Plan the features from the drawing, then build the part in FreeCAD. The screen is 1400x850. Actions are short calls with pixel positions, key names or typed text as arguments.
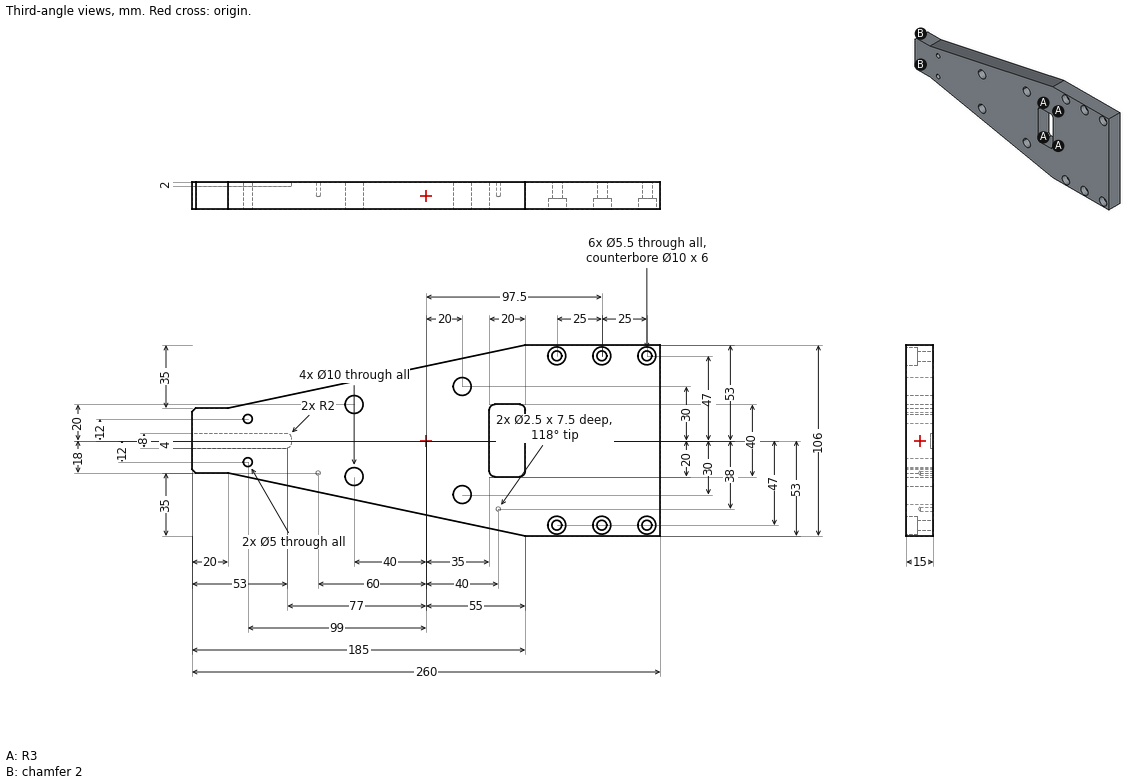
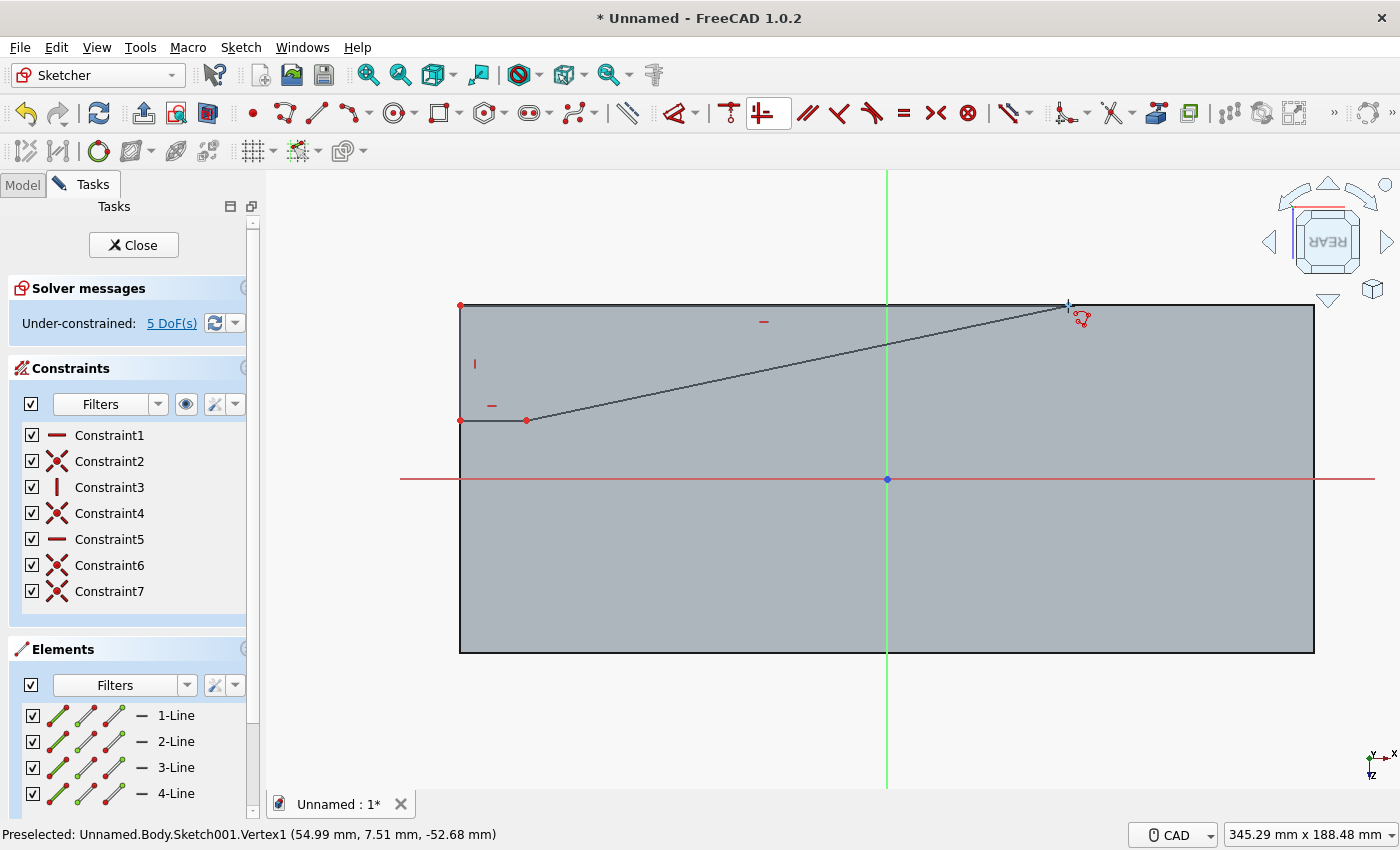
click(1068, 653)
click(526, 538)
click(460, 538)
click(460, 653)
click(1068, 654)
key(Escape)
key(Escape)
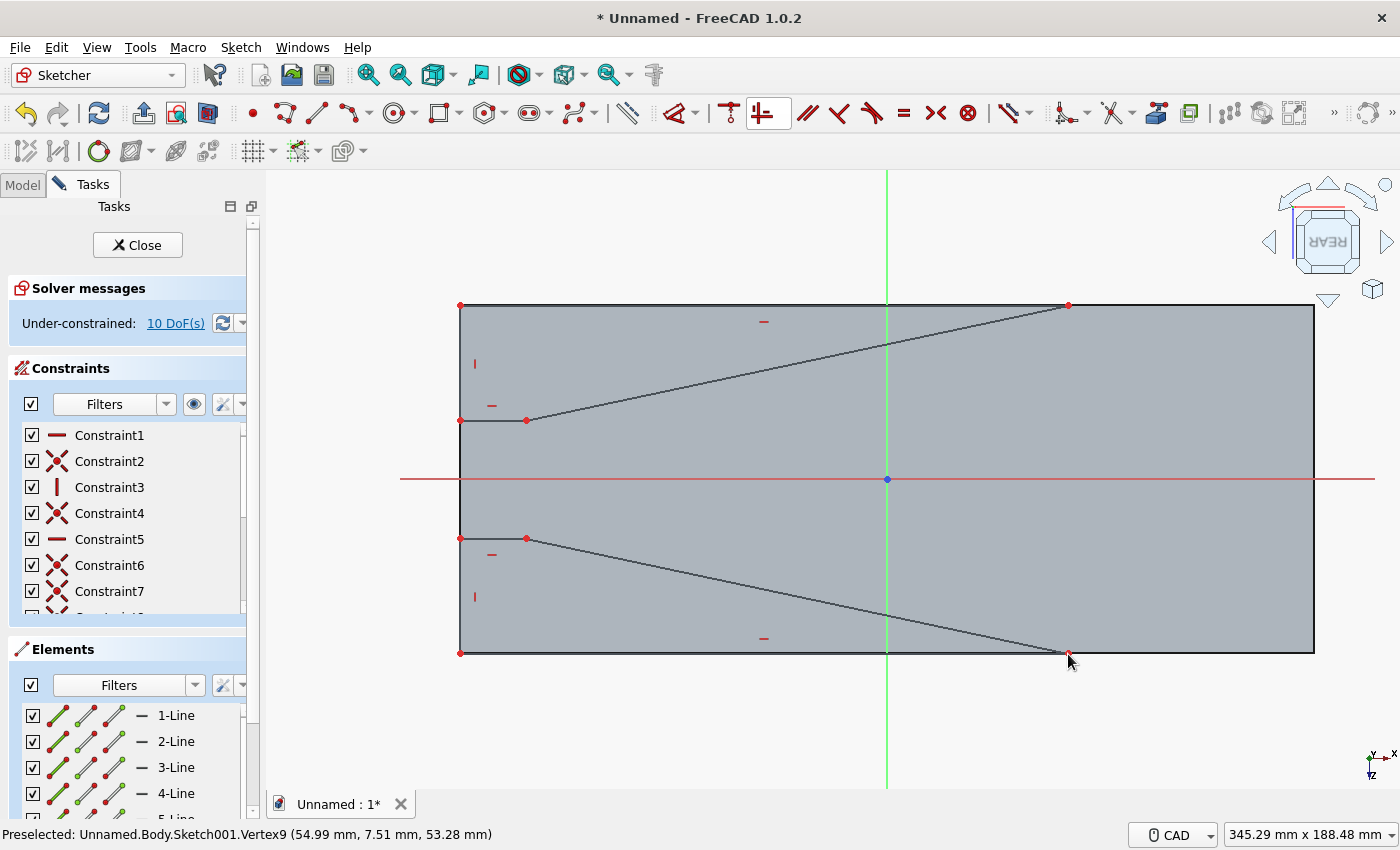
key(d)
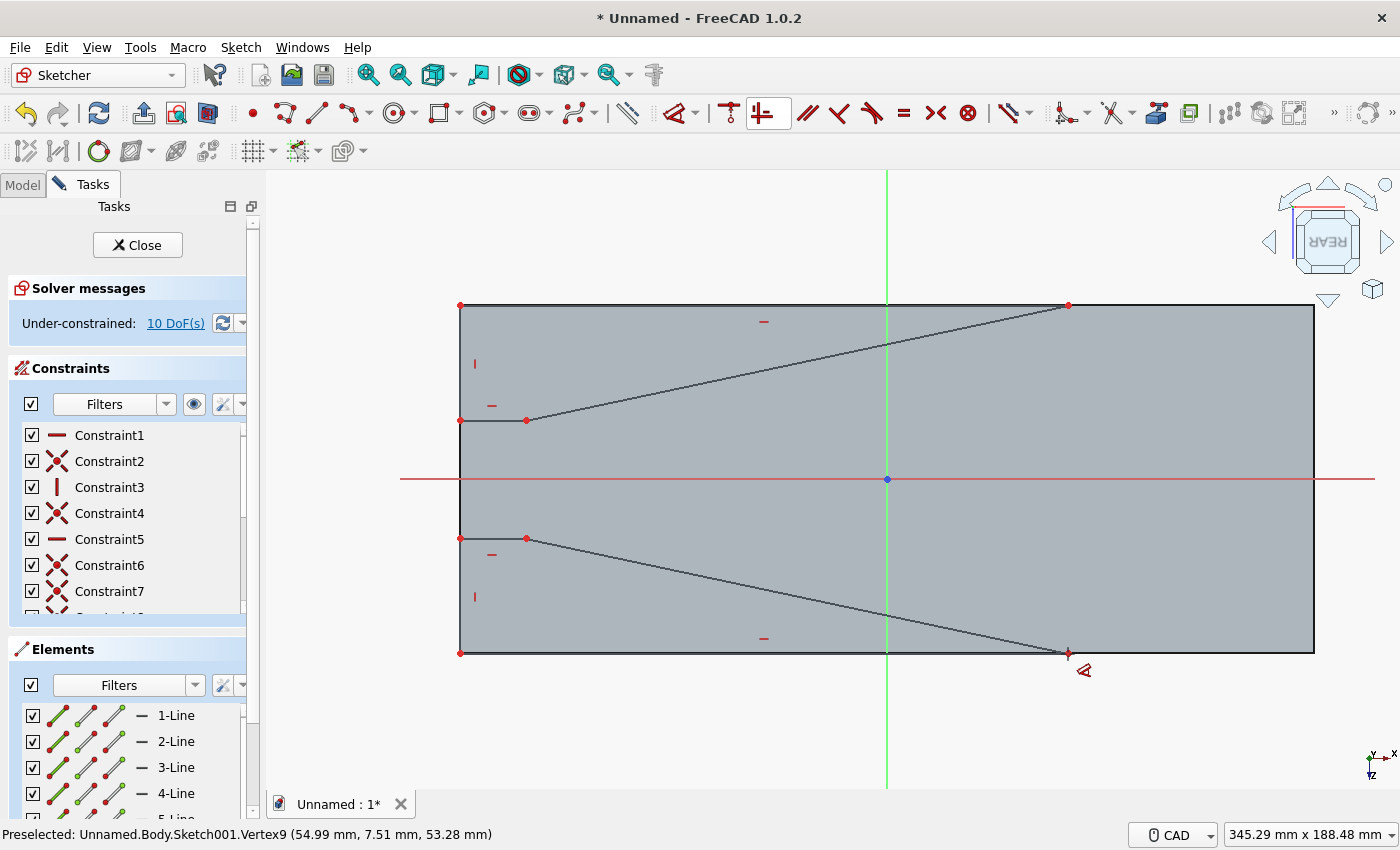
click(460, 341)
click(426, 364)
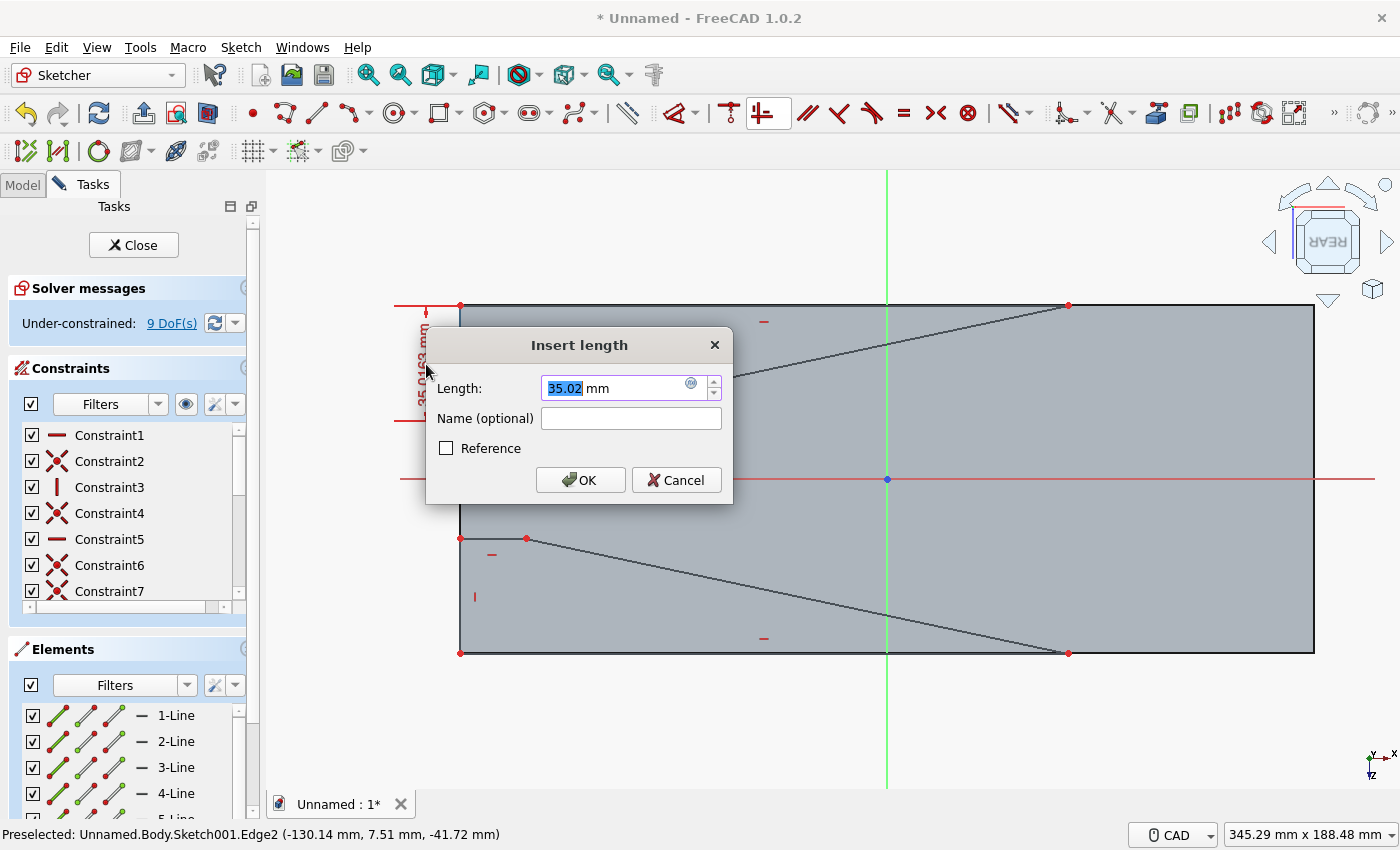
text(35)
key(Return)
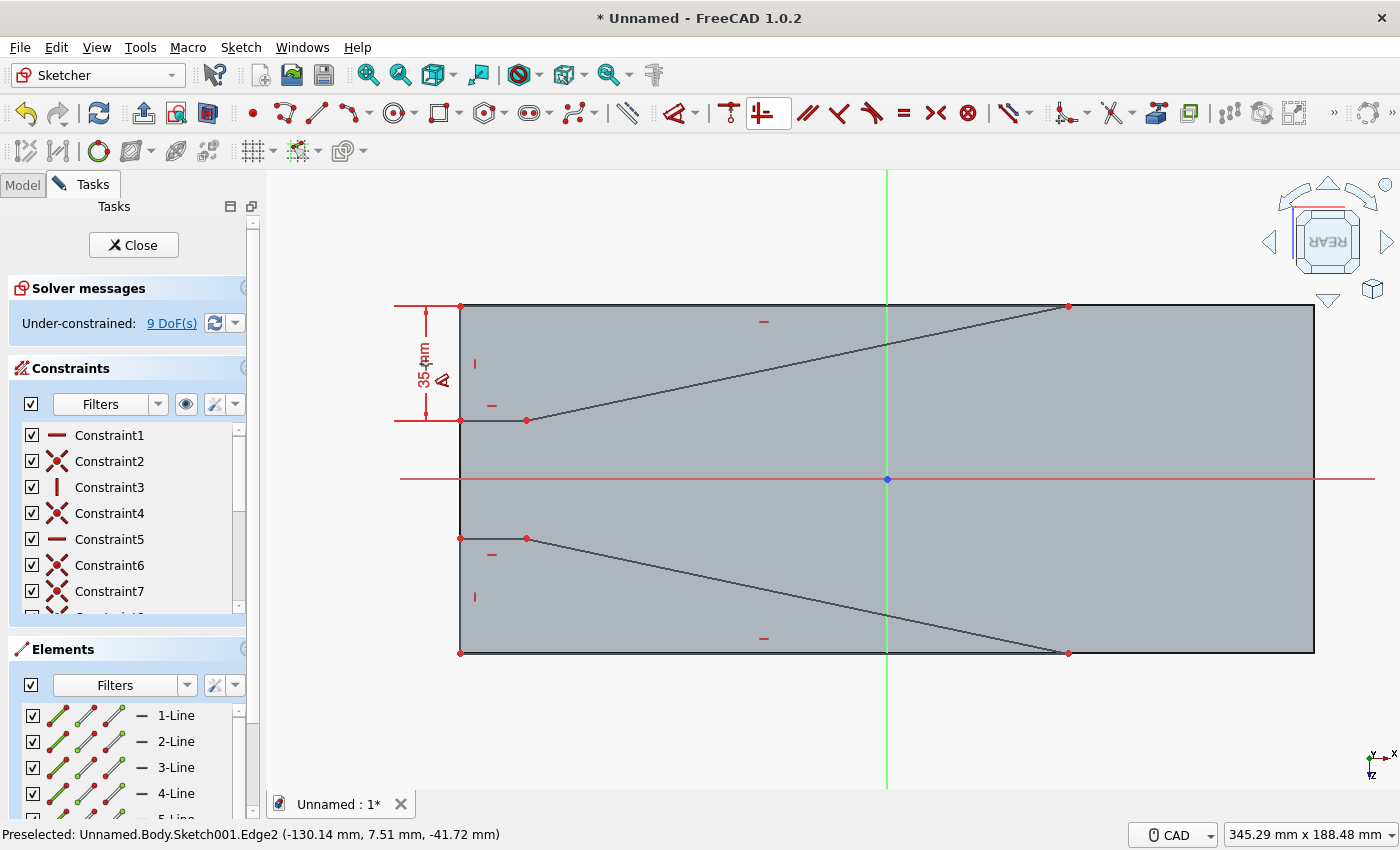
click(480, 421)
click(493, 387)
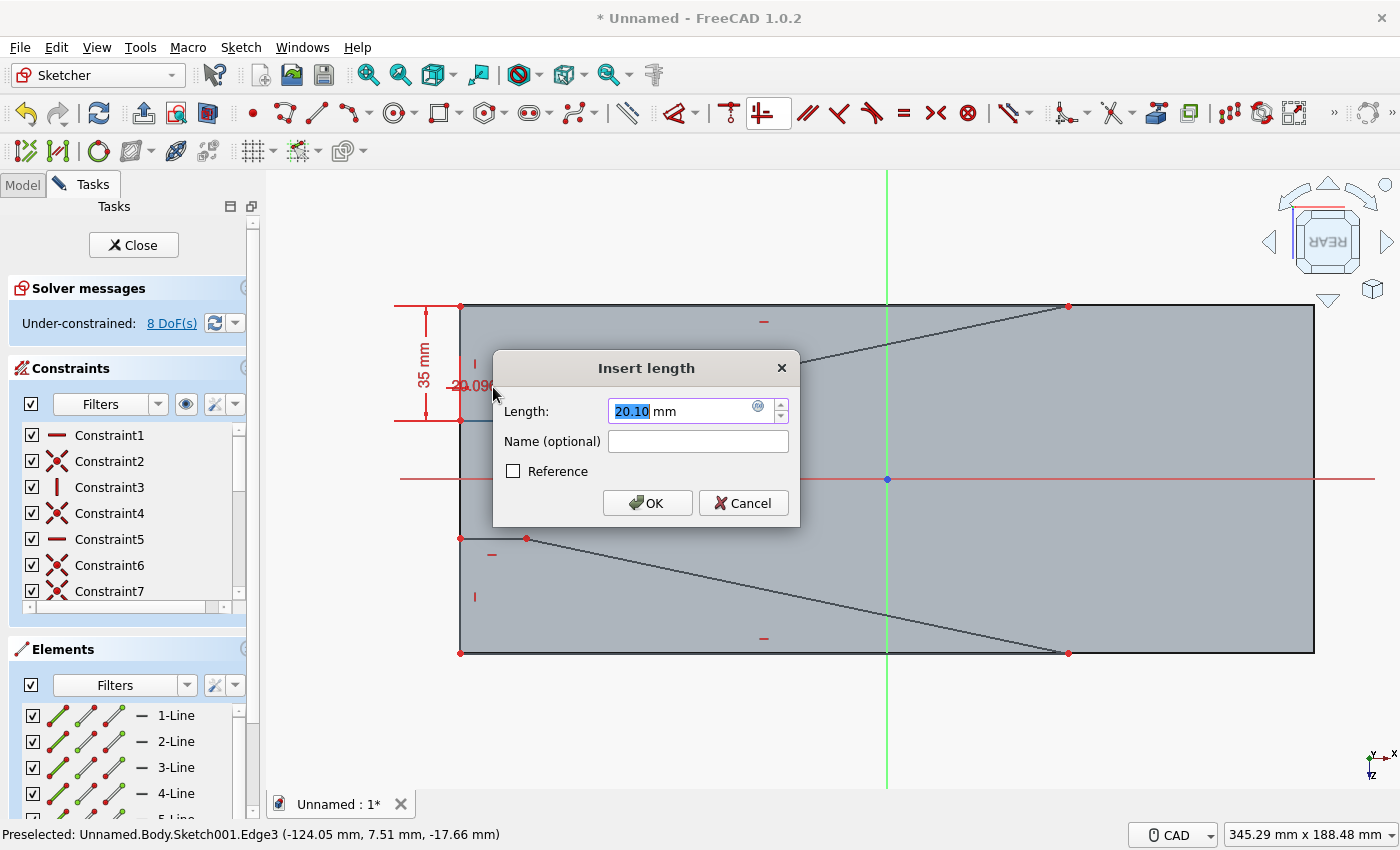
text(20)
key(Return)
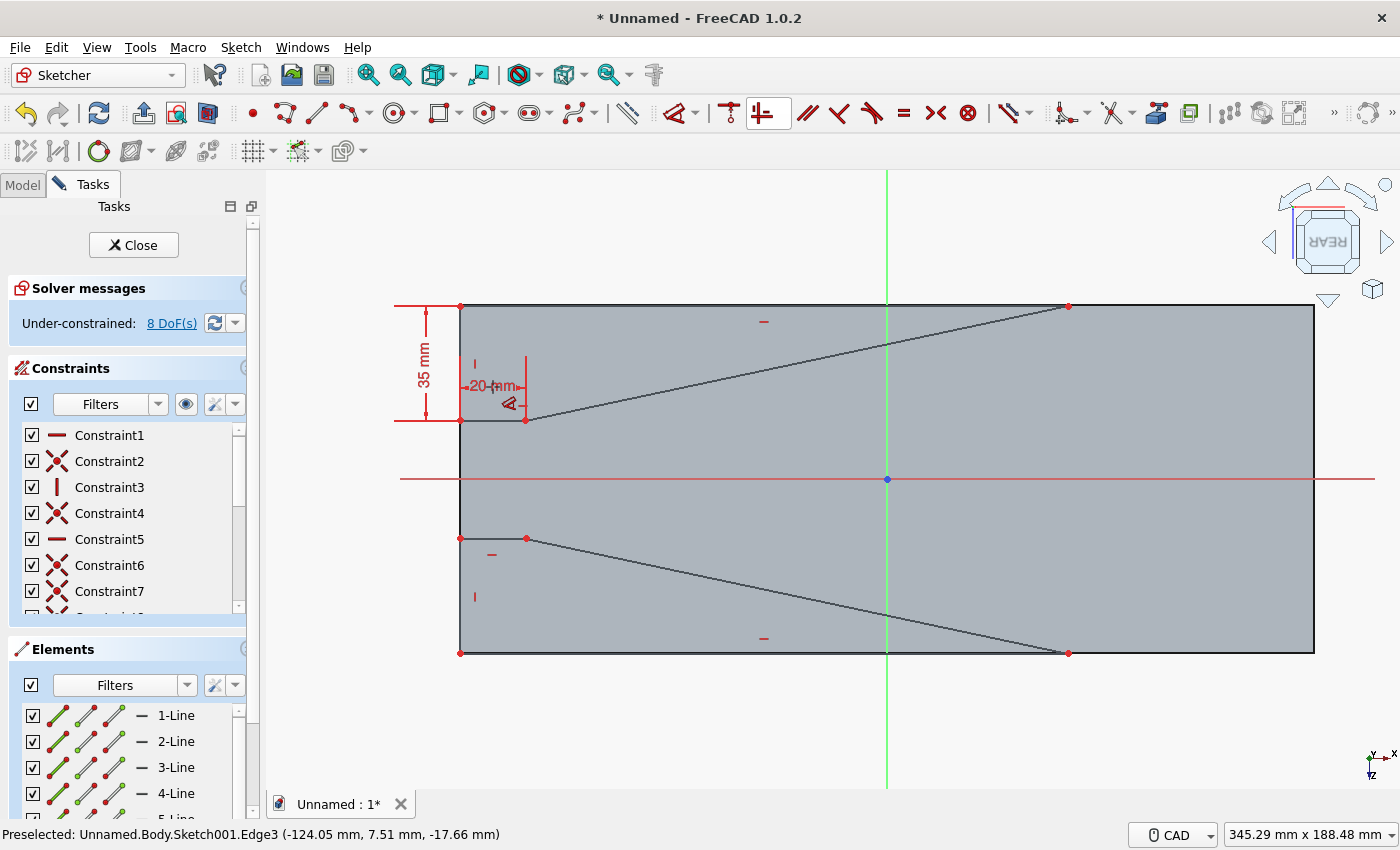
click(506, 539)
click(493, 573)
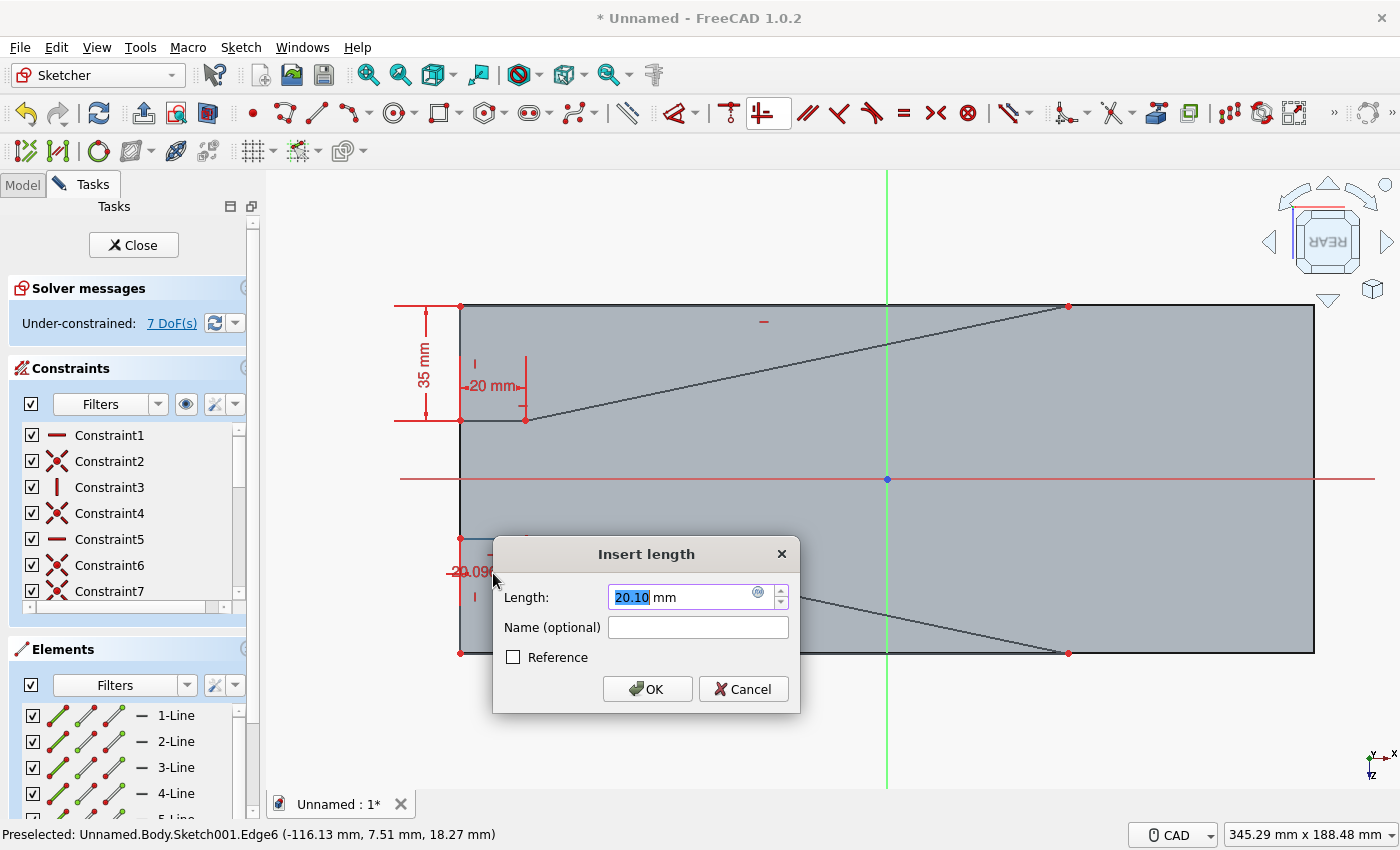
text(20)
key(Return)